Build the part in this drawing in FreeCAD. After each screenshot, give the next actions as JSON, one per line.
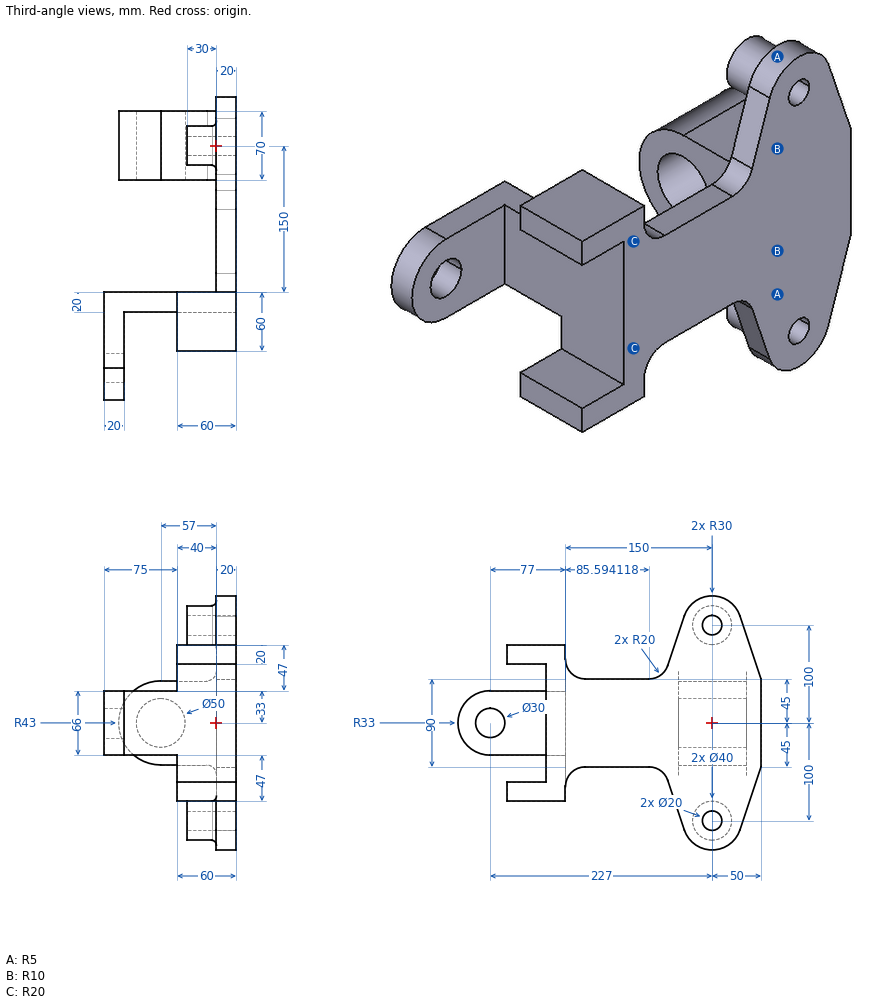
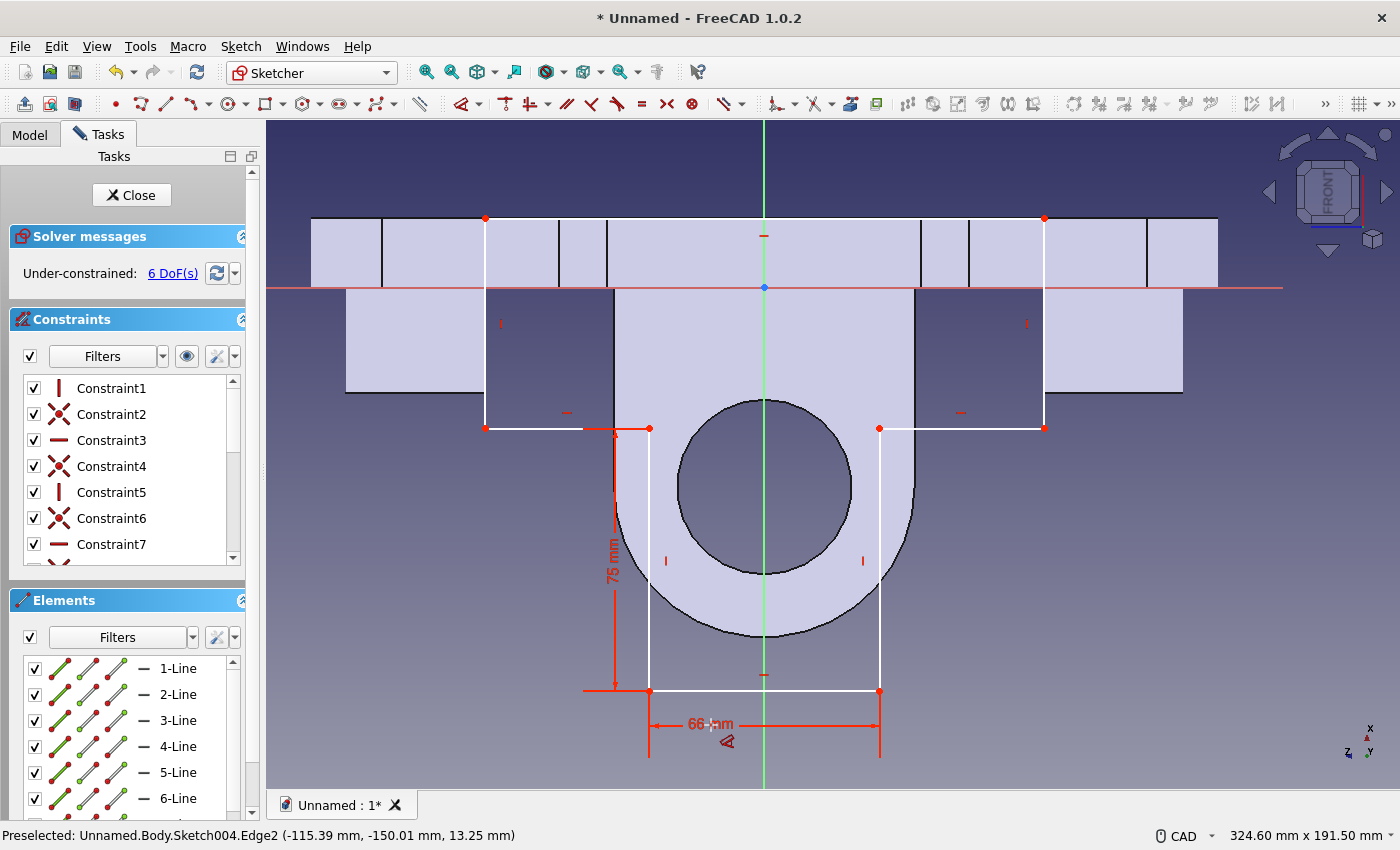
{"action": "left_click", "coordinate": [880, 612]}
{"action": "left_click", "coordinate": [914, 560]}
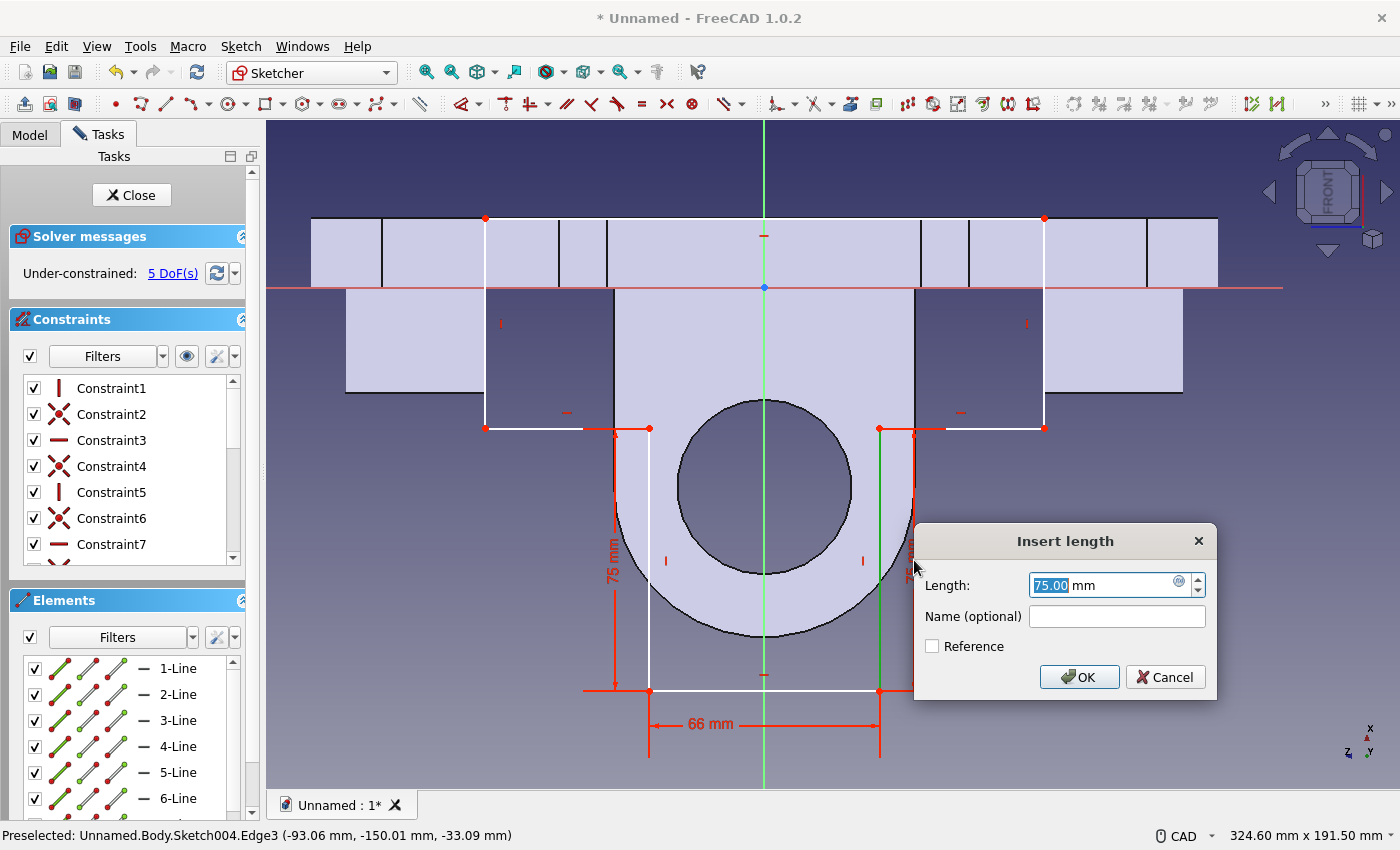
{"action": "type", "text": "75"}
{"action": "key", "text": "Return"}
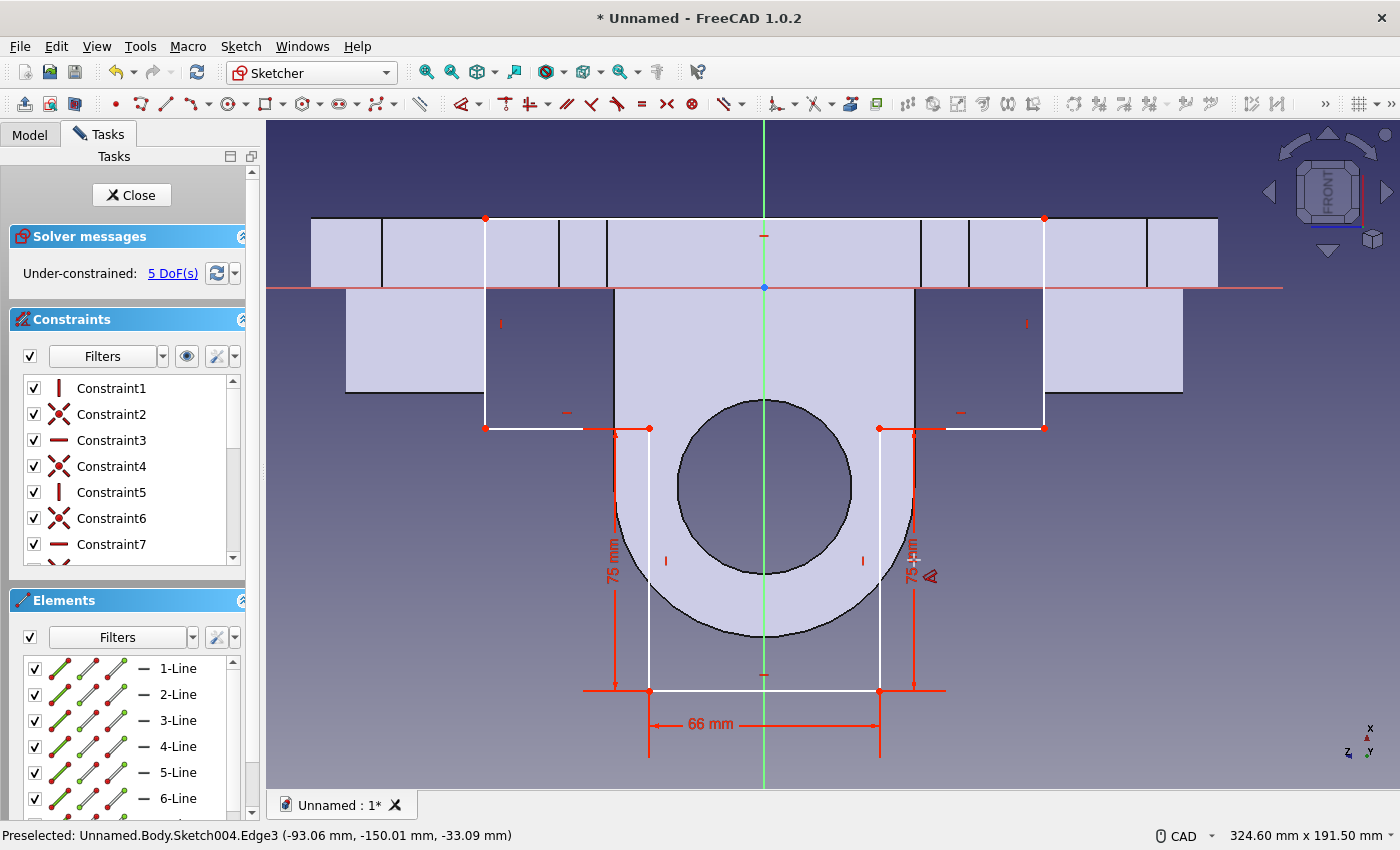
{"action": "left_click", "coordinate": [929, 429]}
{"action": "left_click", "coordinate": [962, 395]}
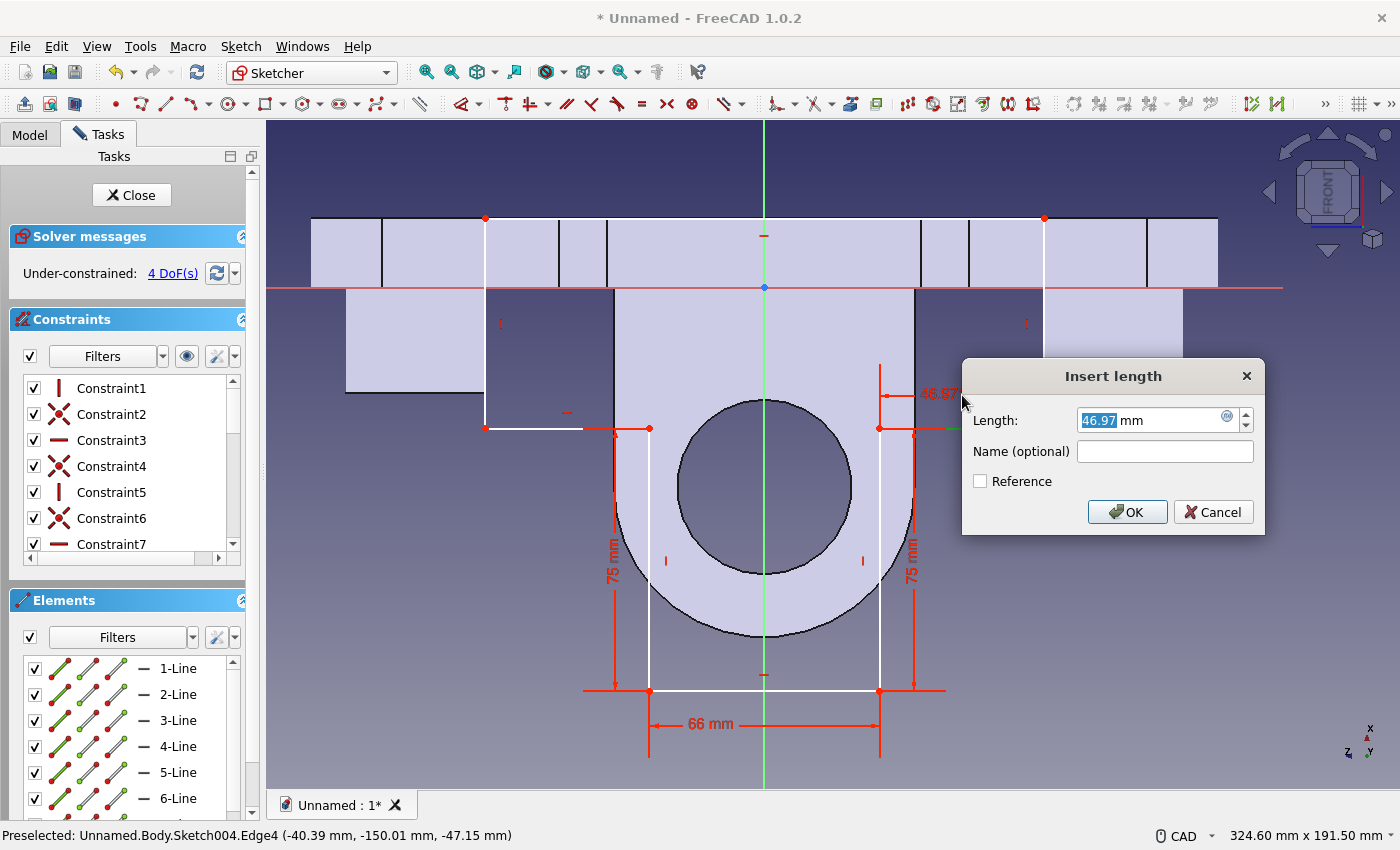
{"action": "type", "text": "47"}
{"action": "key", "text": "Return"}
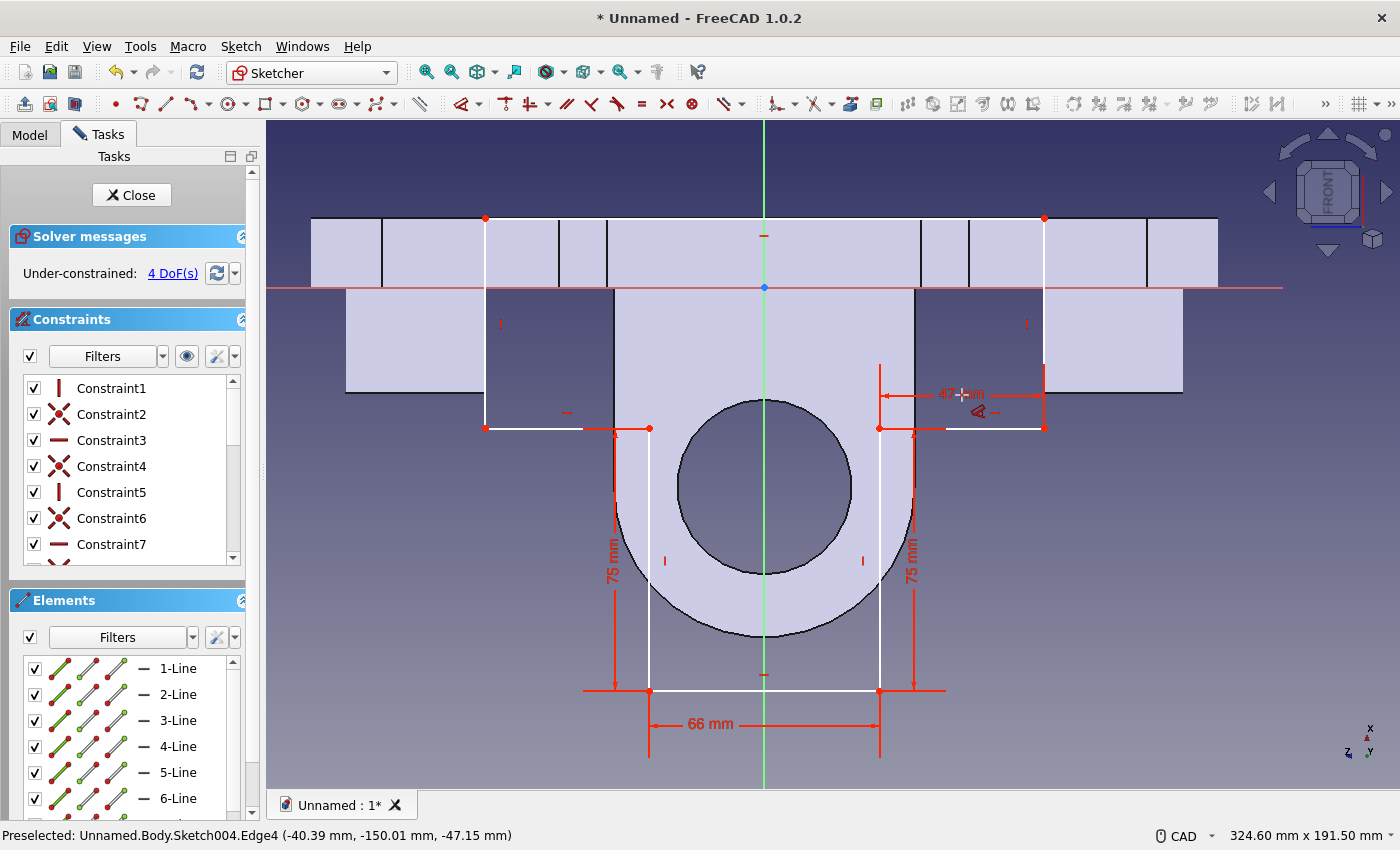
{"action": "left_click", "coordinate": [1044, 366]}
{"action": "left_click", "coordinate": [1078, 324]}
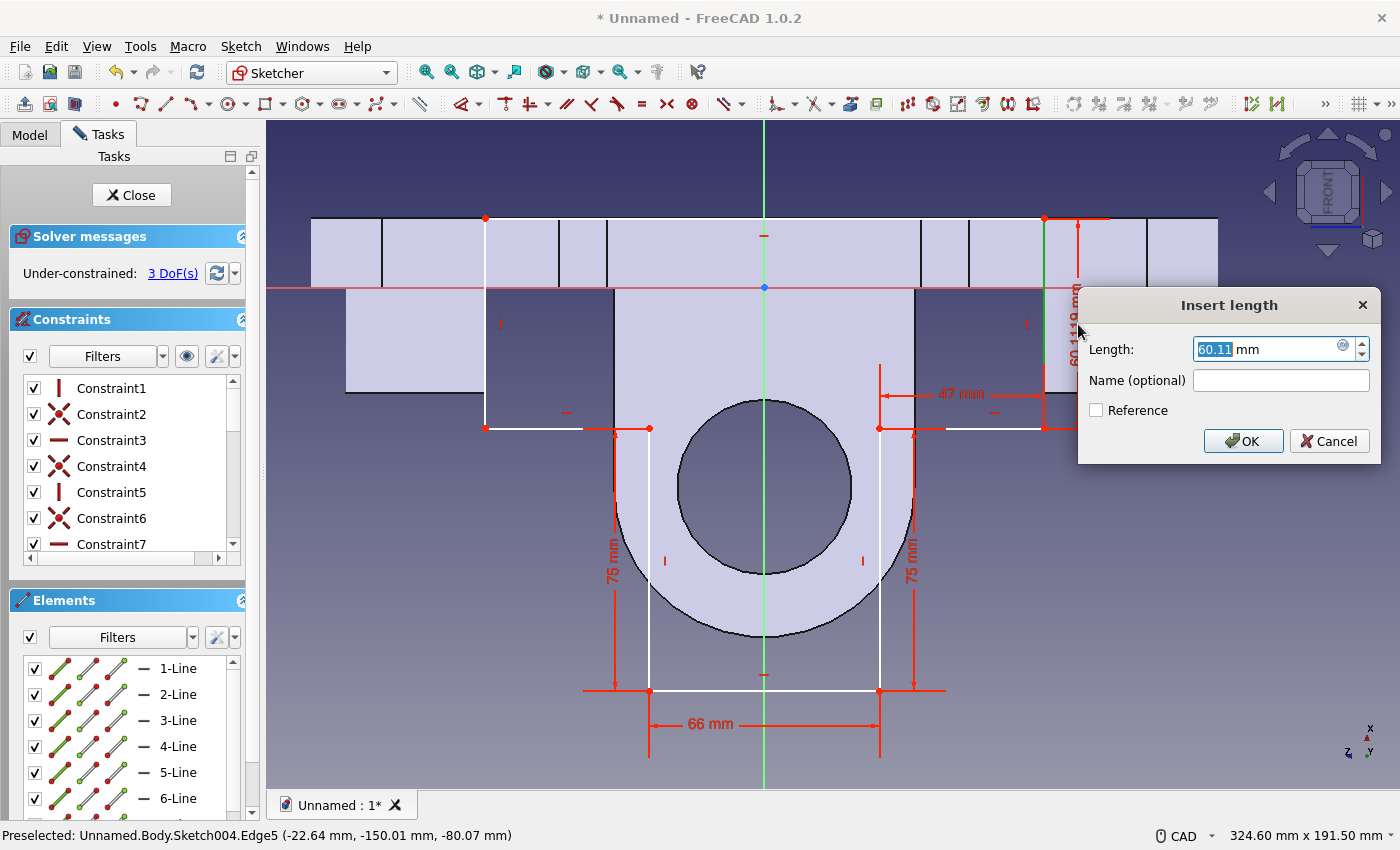
{"action": "type", "text": "60"}
{"action": "key", "text": "Return"}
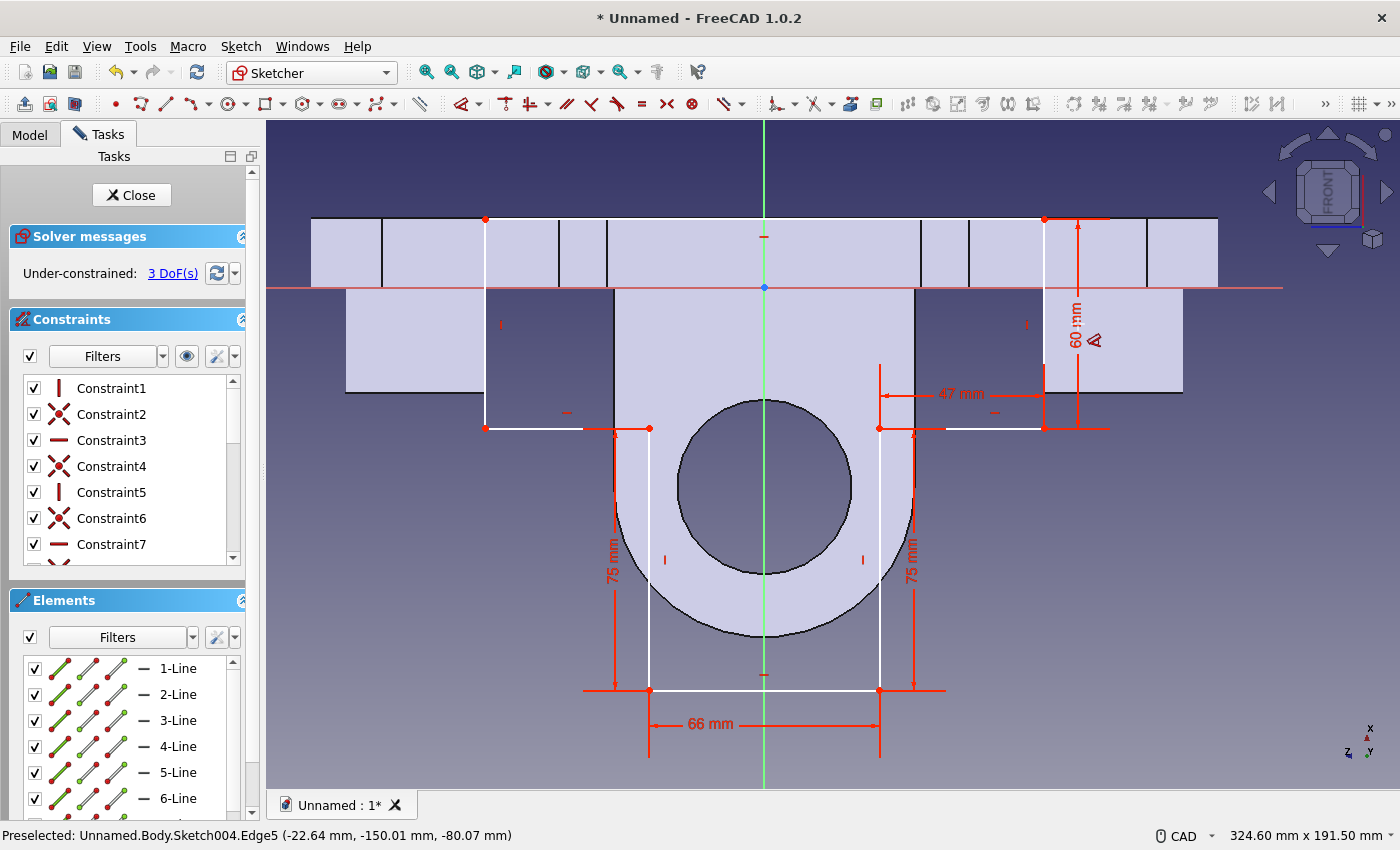
{"action": "left_click", "coordinate": [534, 429]}
{"action": "left_click", "coordinate": [567, 395]}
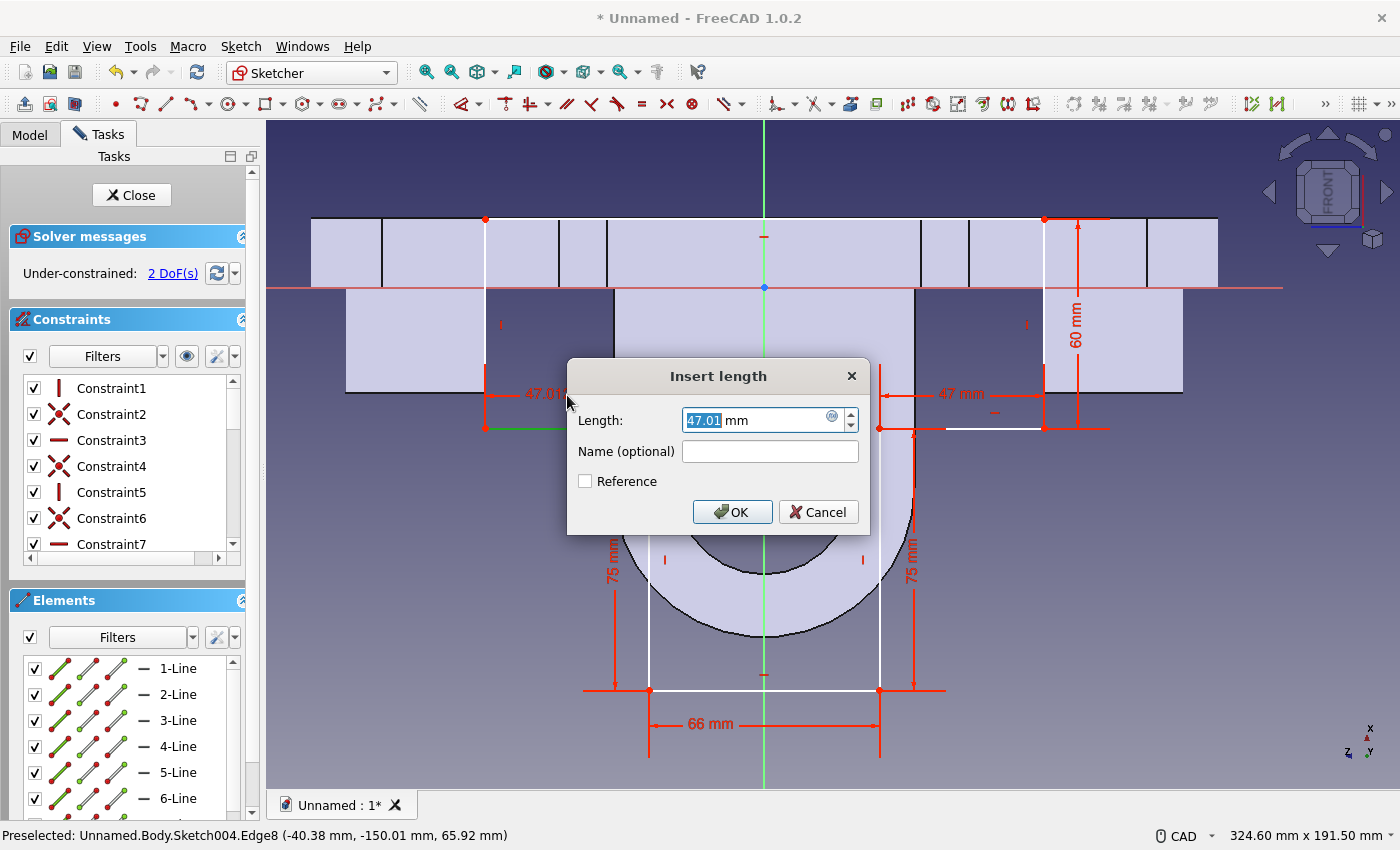
{"action": "type", "text": "47"}
{"action": "key", "text": "Return"}